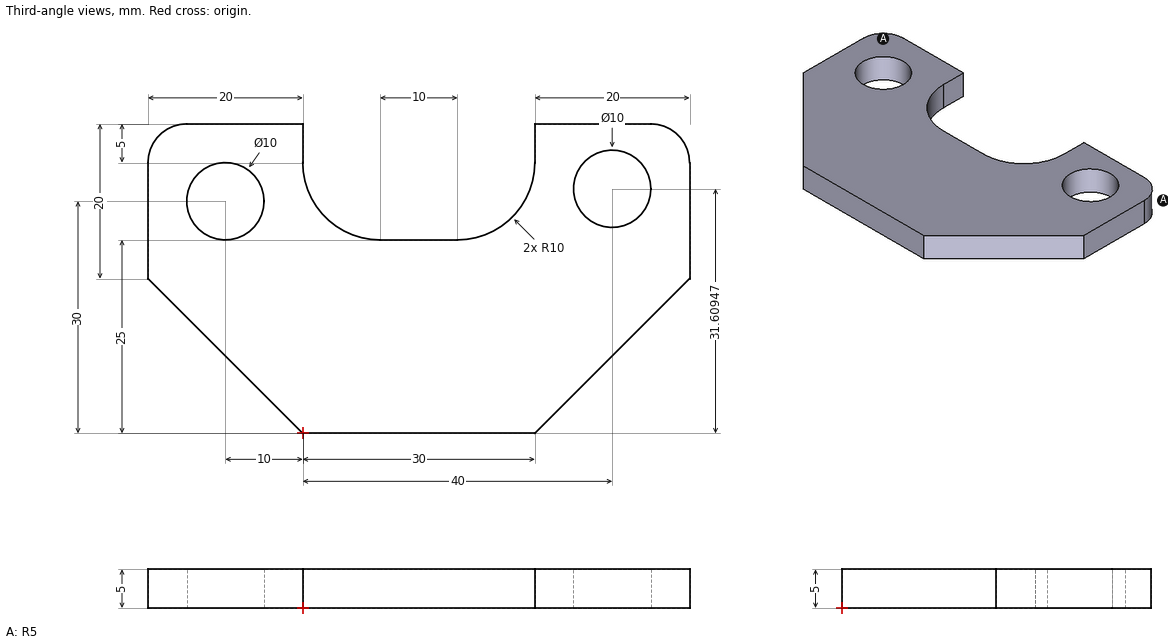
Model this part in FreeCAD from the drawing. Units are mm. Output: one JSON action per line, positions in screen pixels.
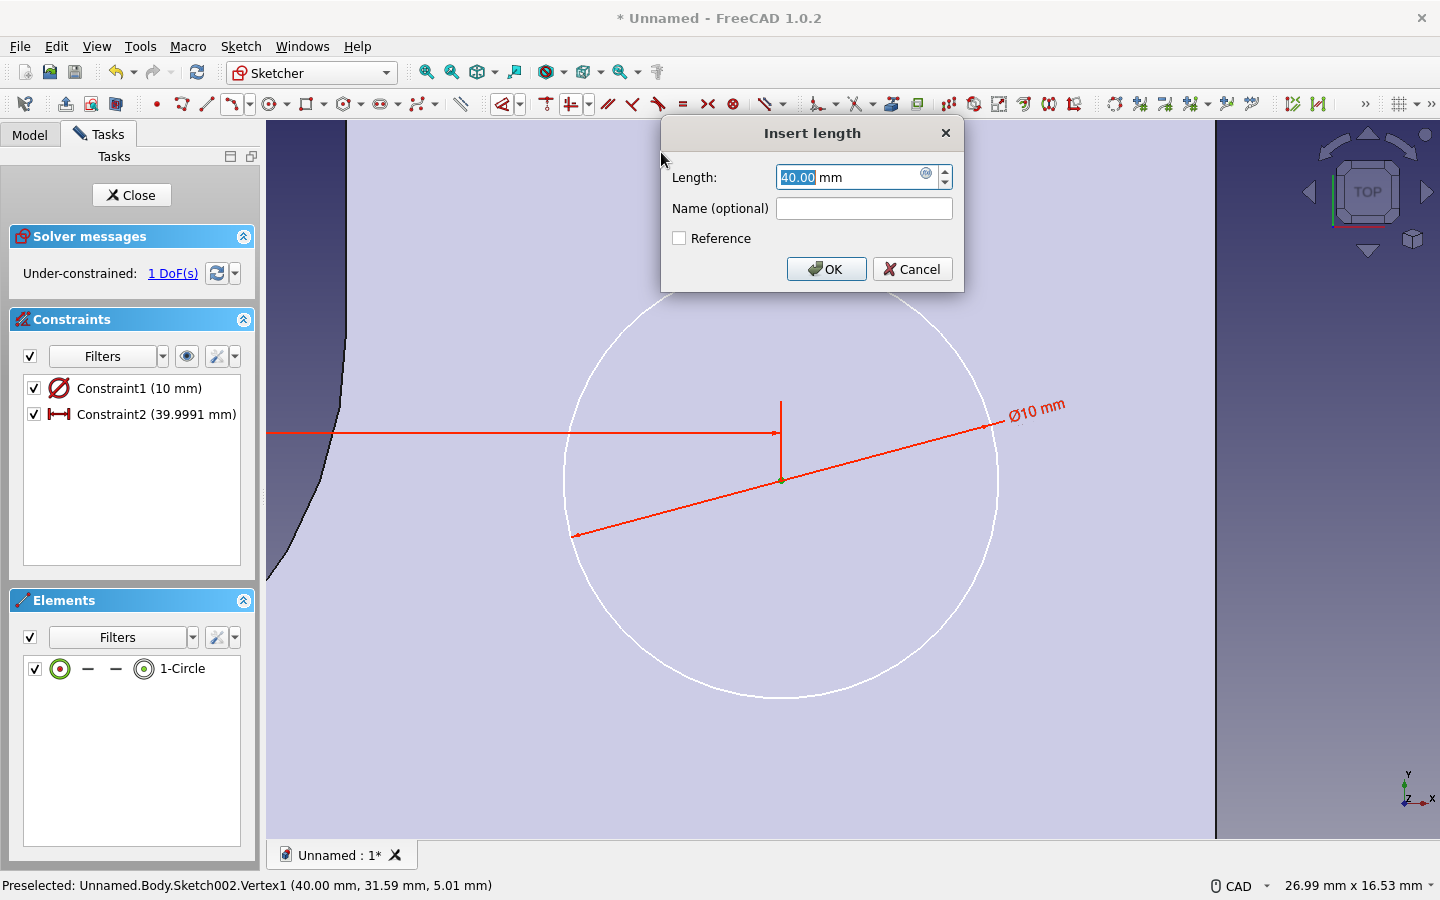
{"action": "type", "text": "40"}
{"action": "key", "text": "Return"}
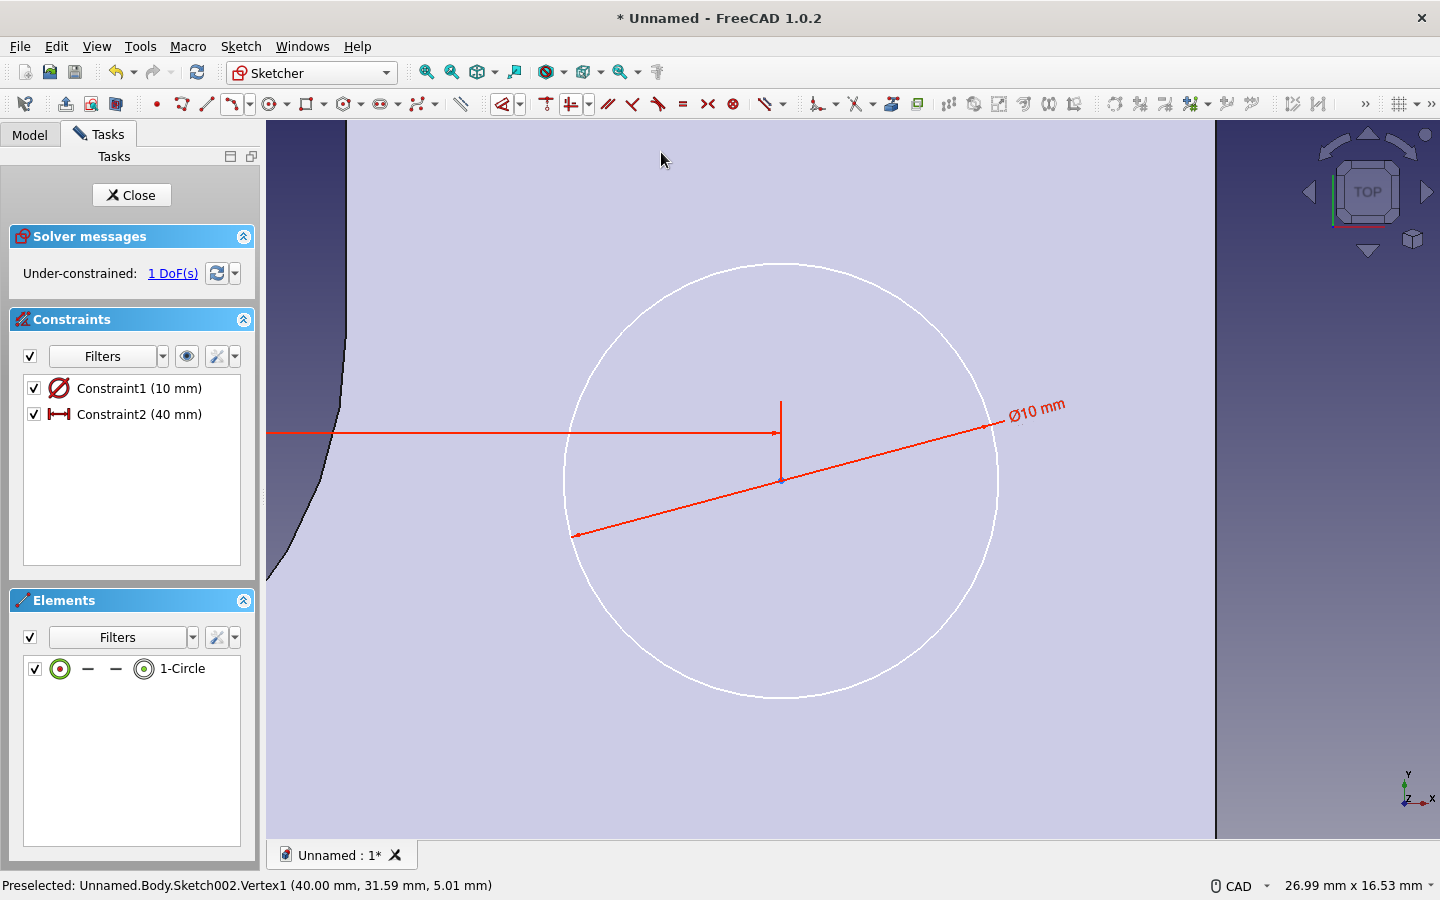
{"action": "left_click", "coordinate": [781, 481]}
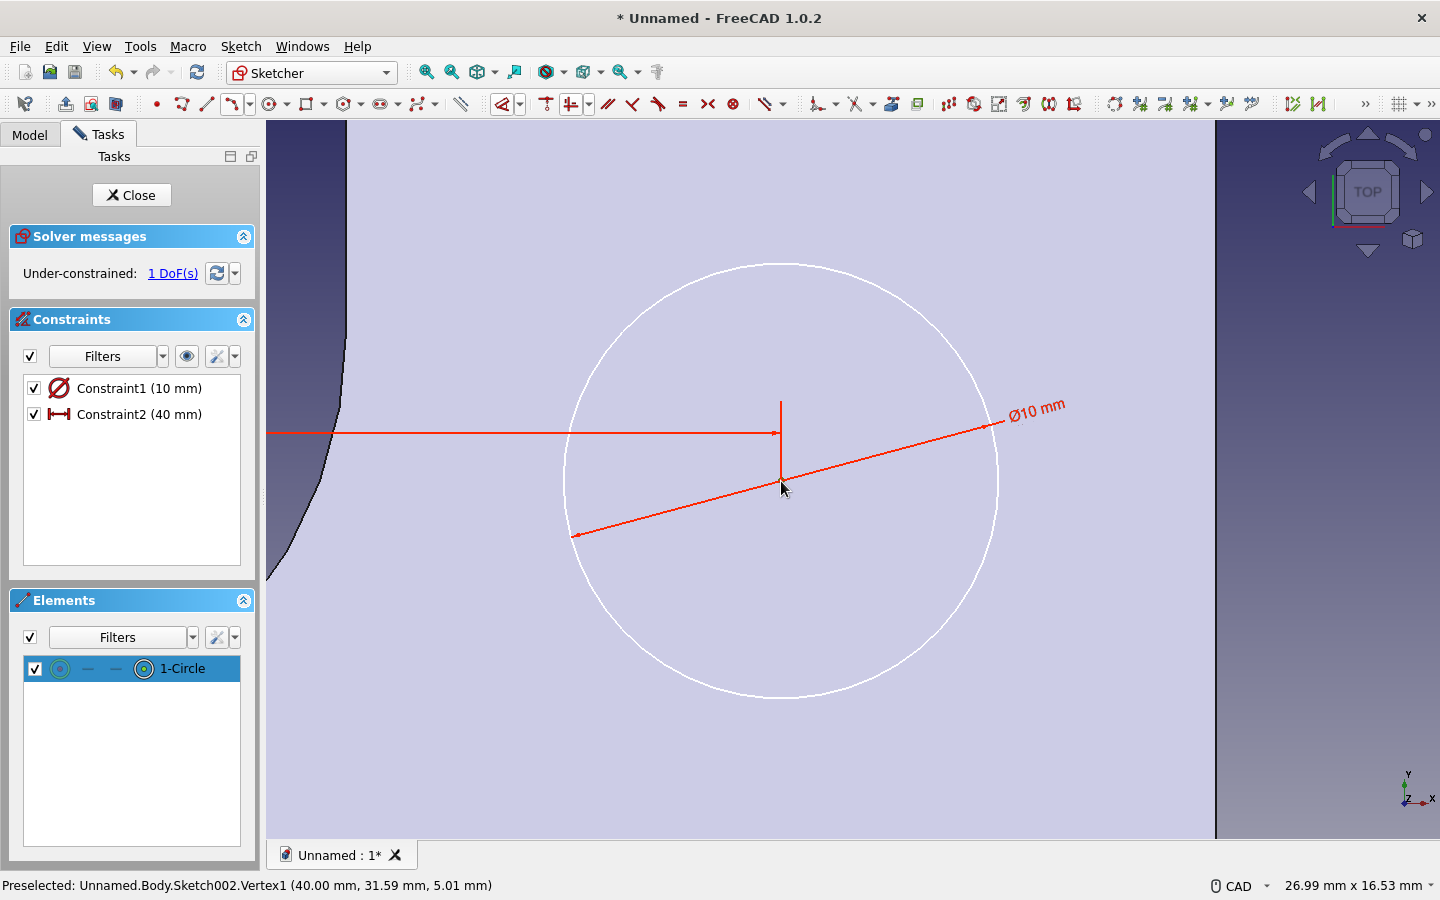
{"action": "key", "text": "i"}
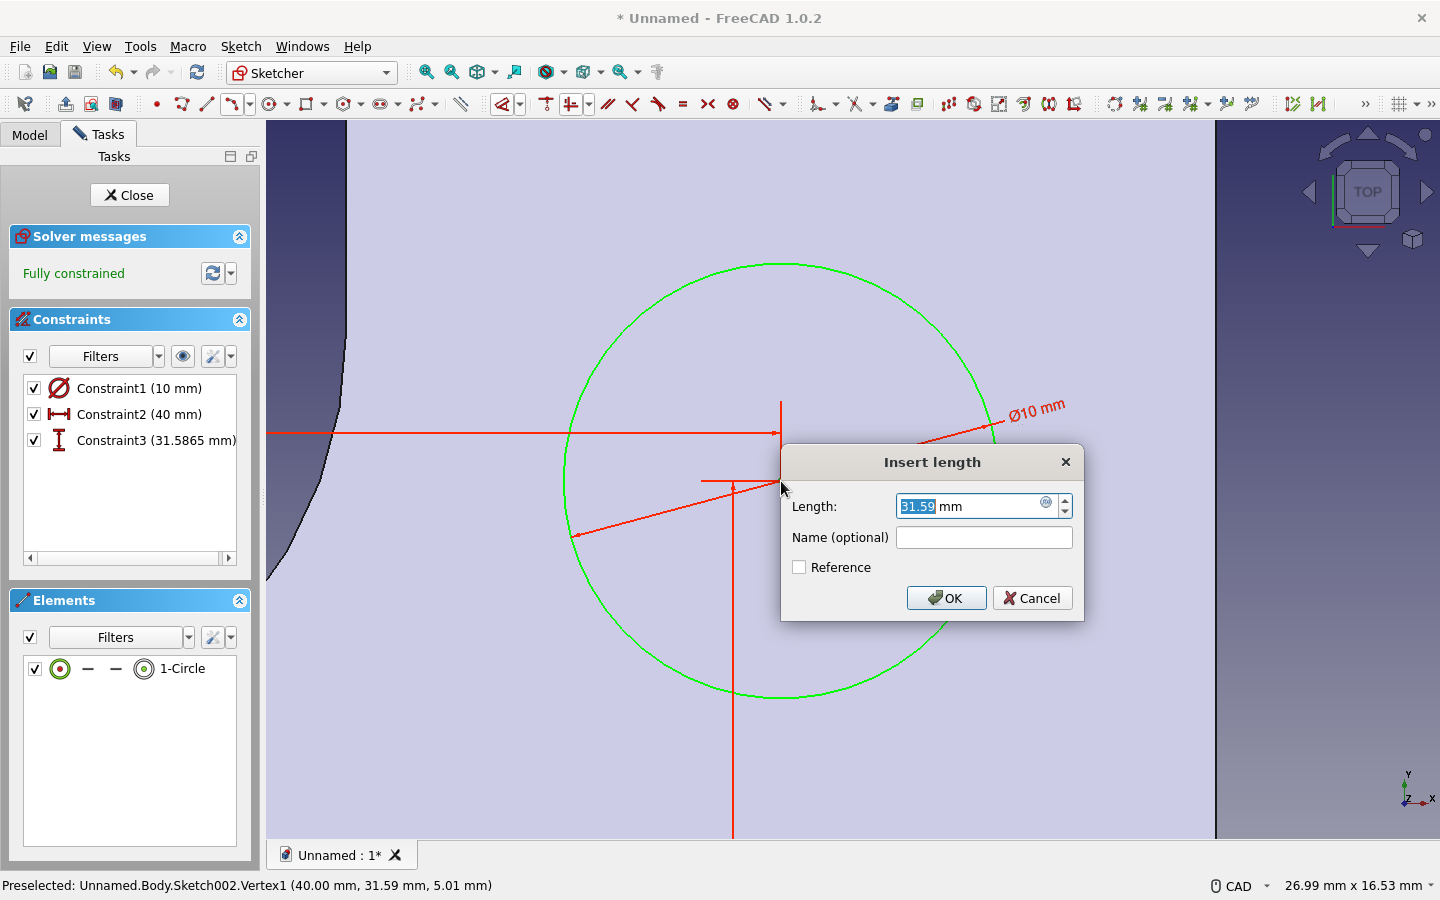
{"action": "type", "text": "31.60947"}
{"action": "key", "text": "Return"}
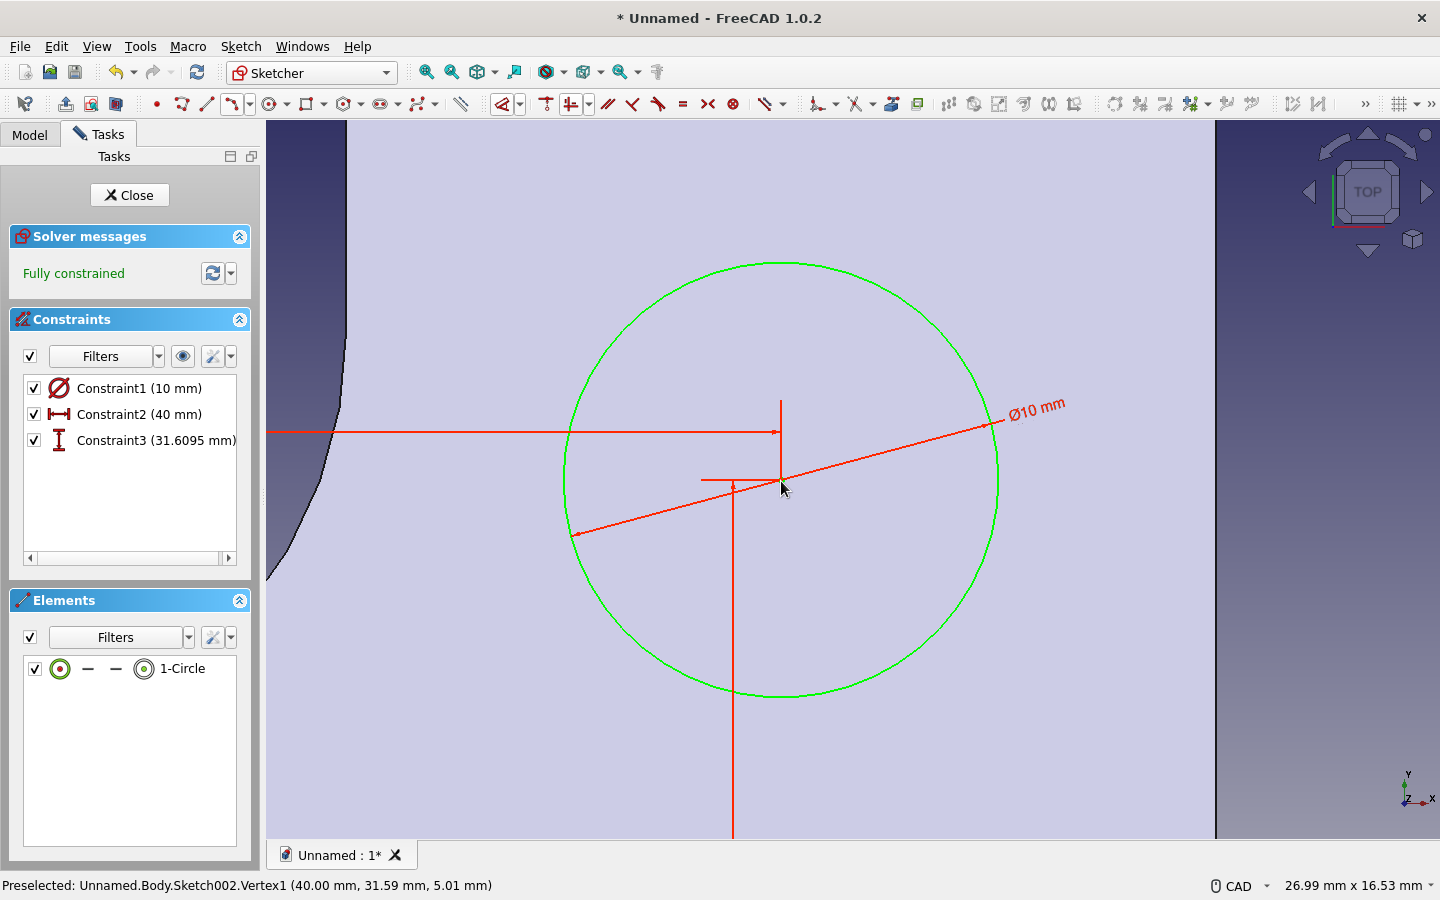
{"action": "left_click", "coordinate": [130, 195]}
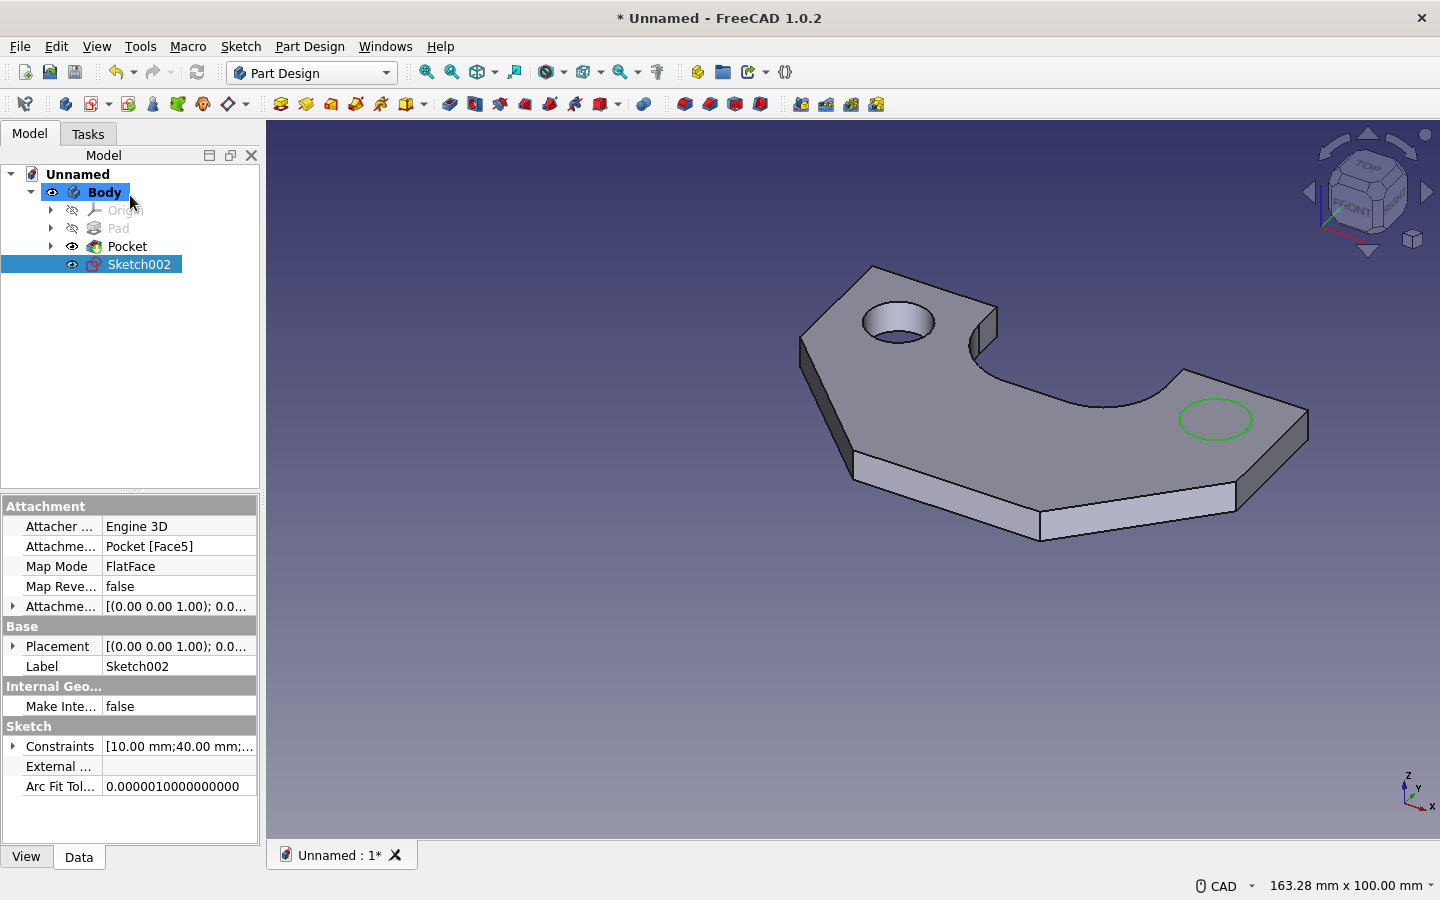
{"action": "left_click", "coordinate": [450, 104]}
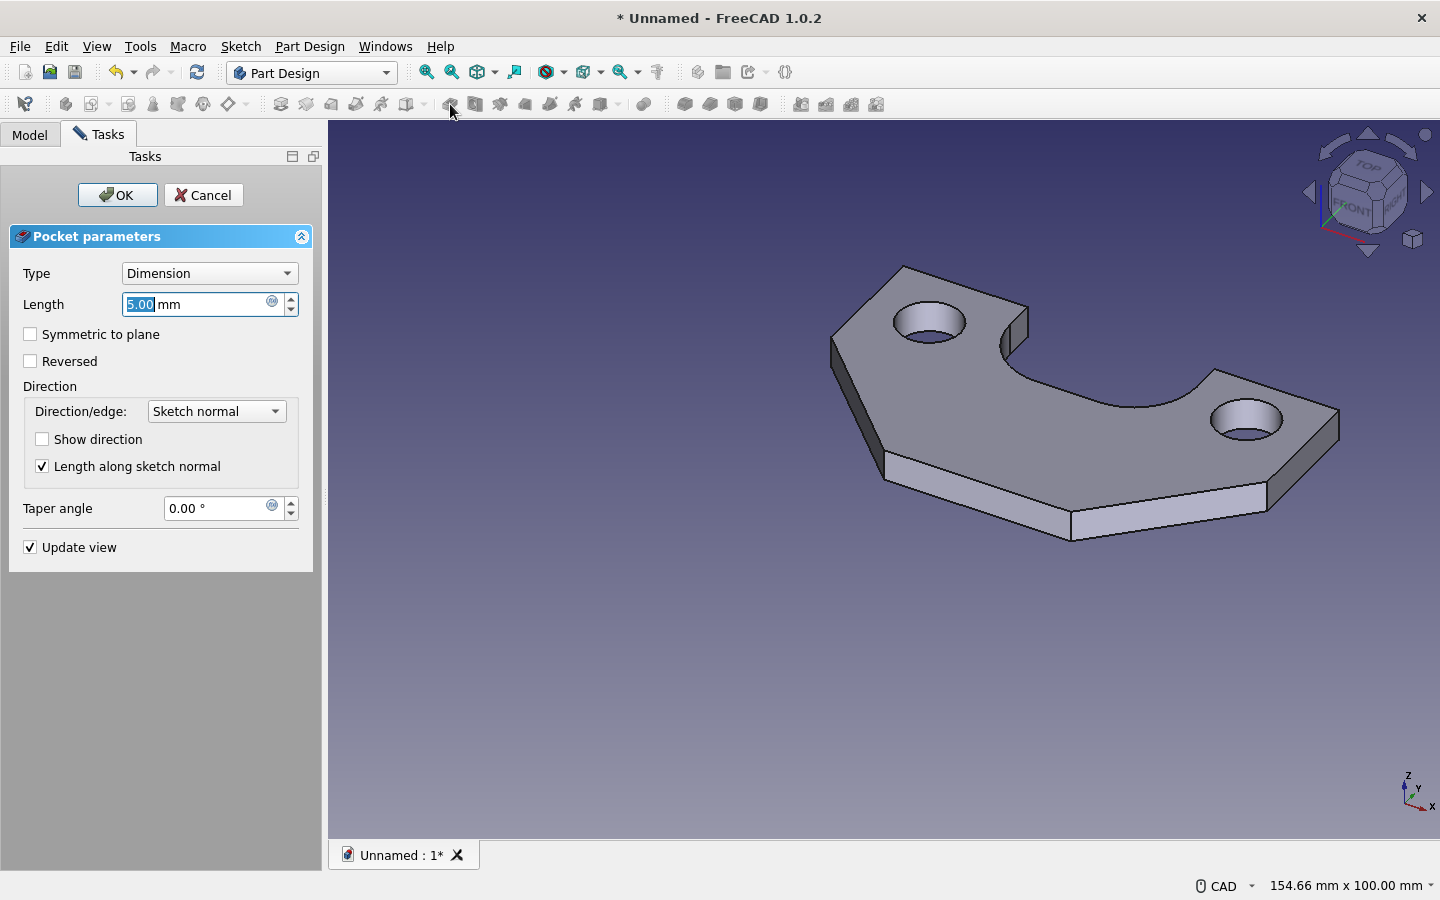
{"action": "type", "text": "5"}
{"action": "key", "text": "Tab"}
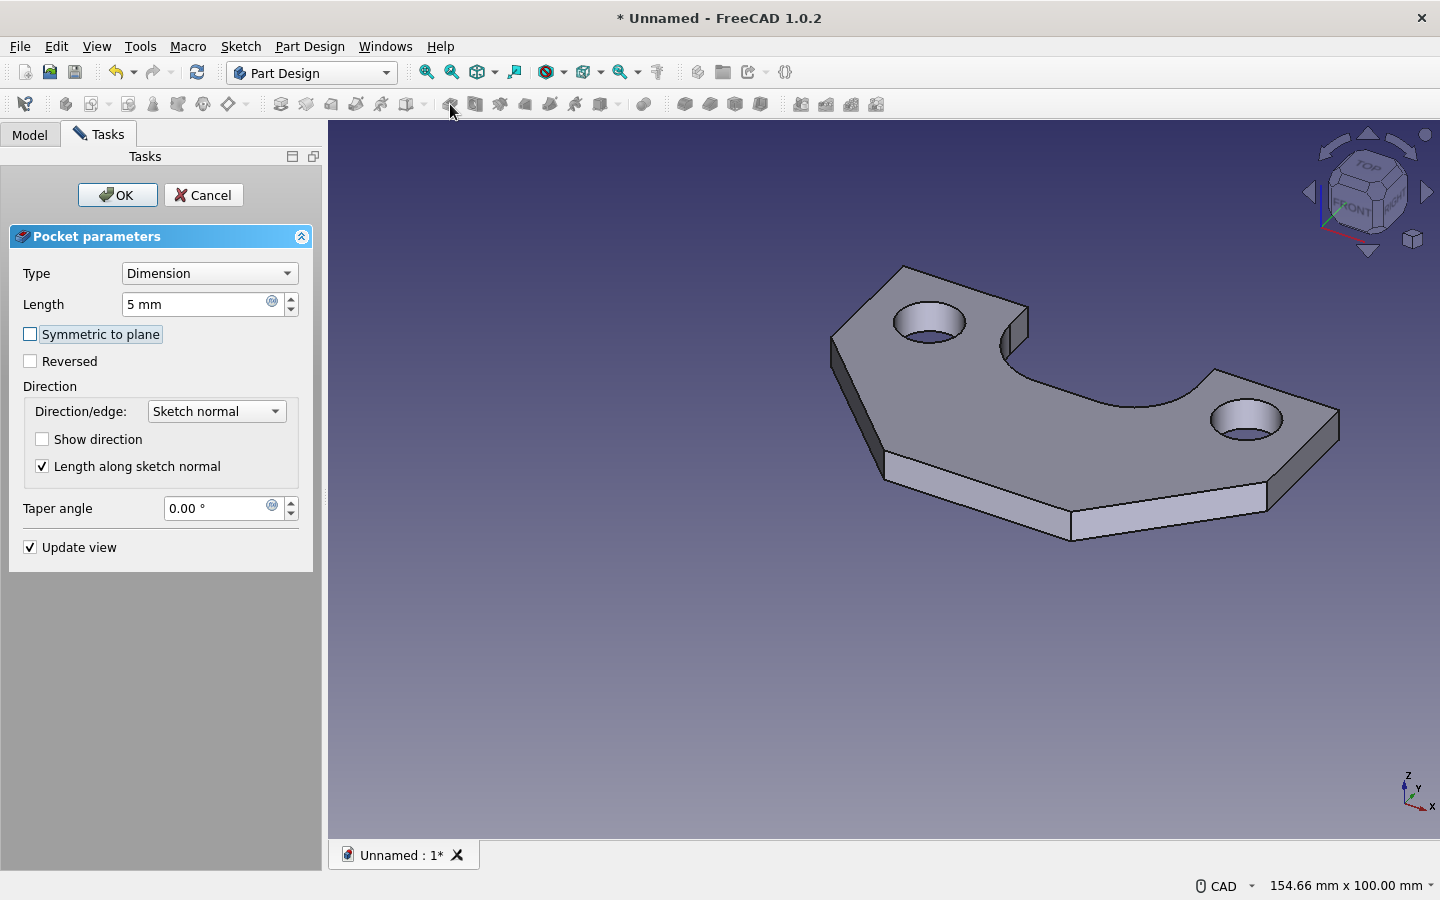
{"action": "left_click", "coordinate": [118, 195]}